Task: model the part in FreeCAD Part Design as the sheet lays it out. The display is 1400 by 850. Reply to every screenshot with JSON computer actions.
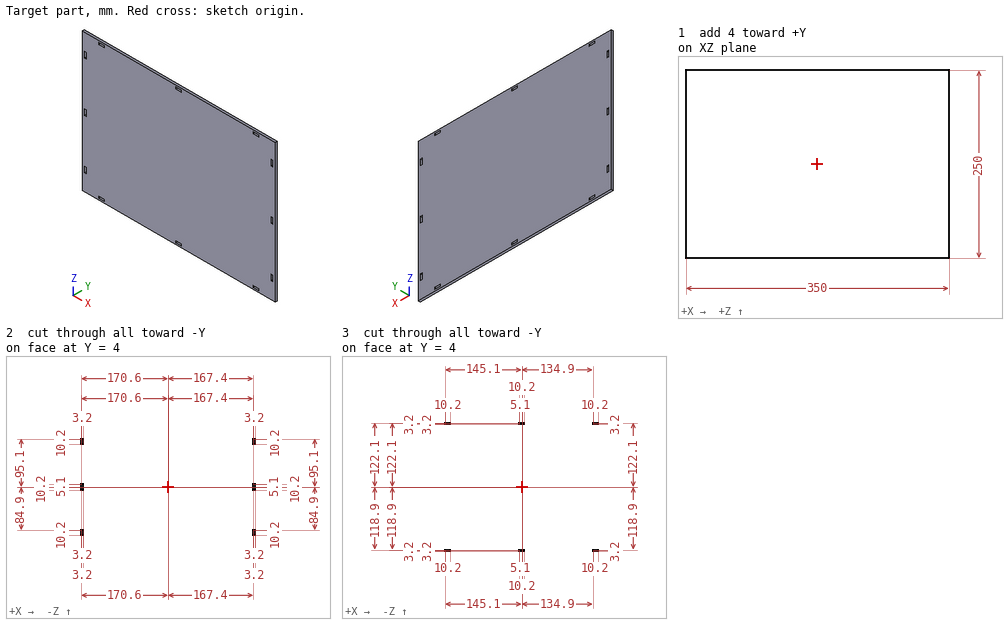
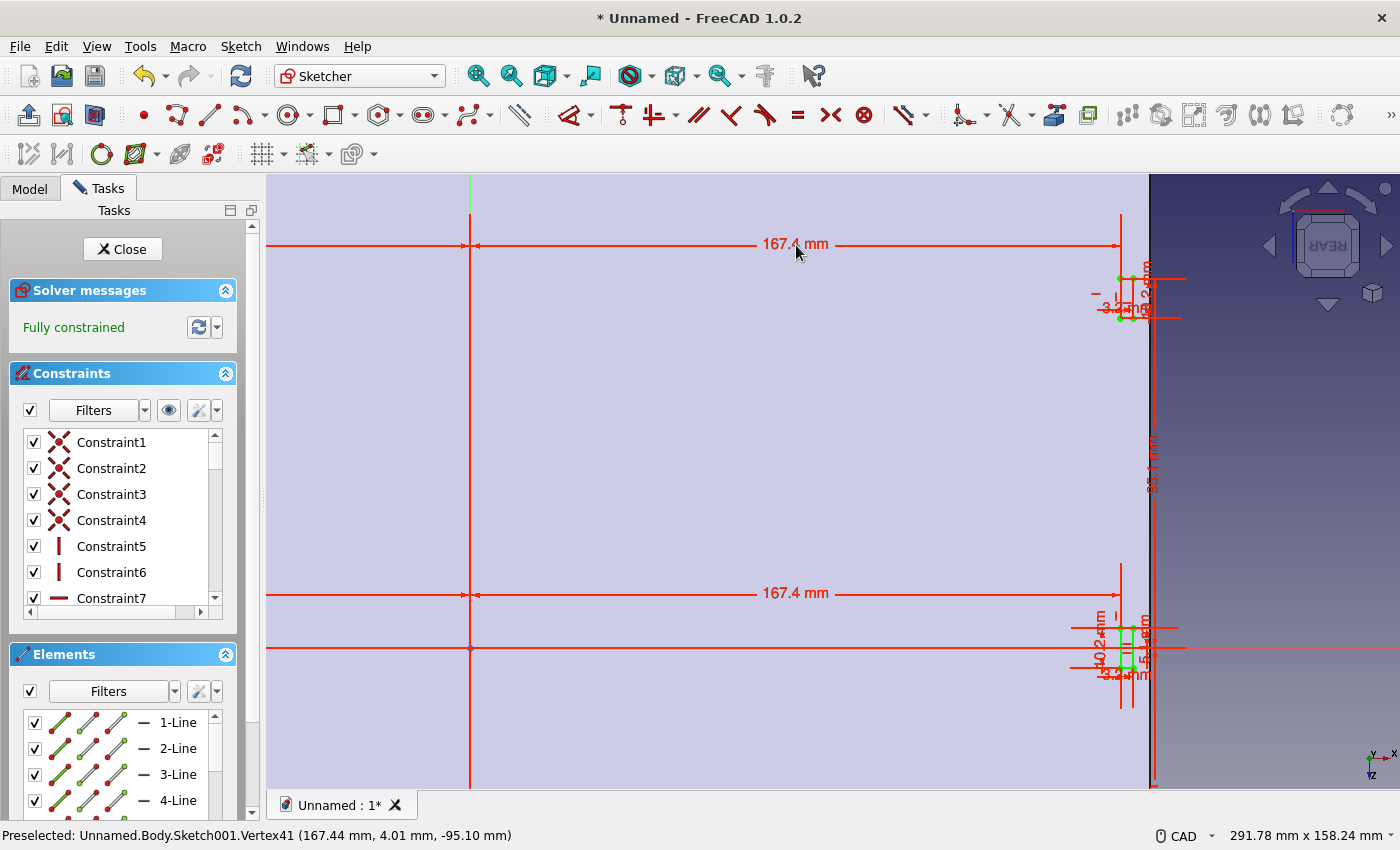
{"action": "left_click", "coordinate": [123, 249]}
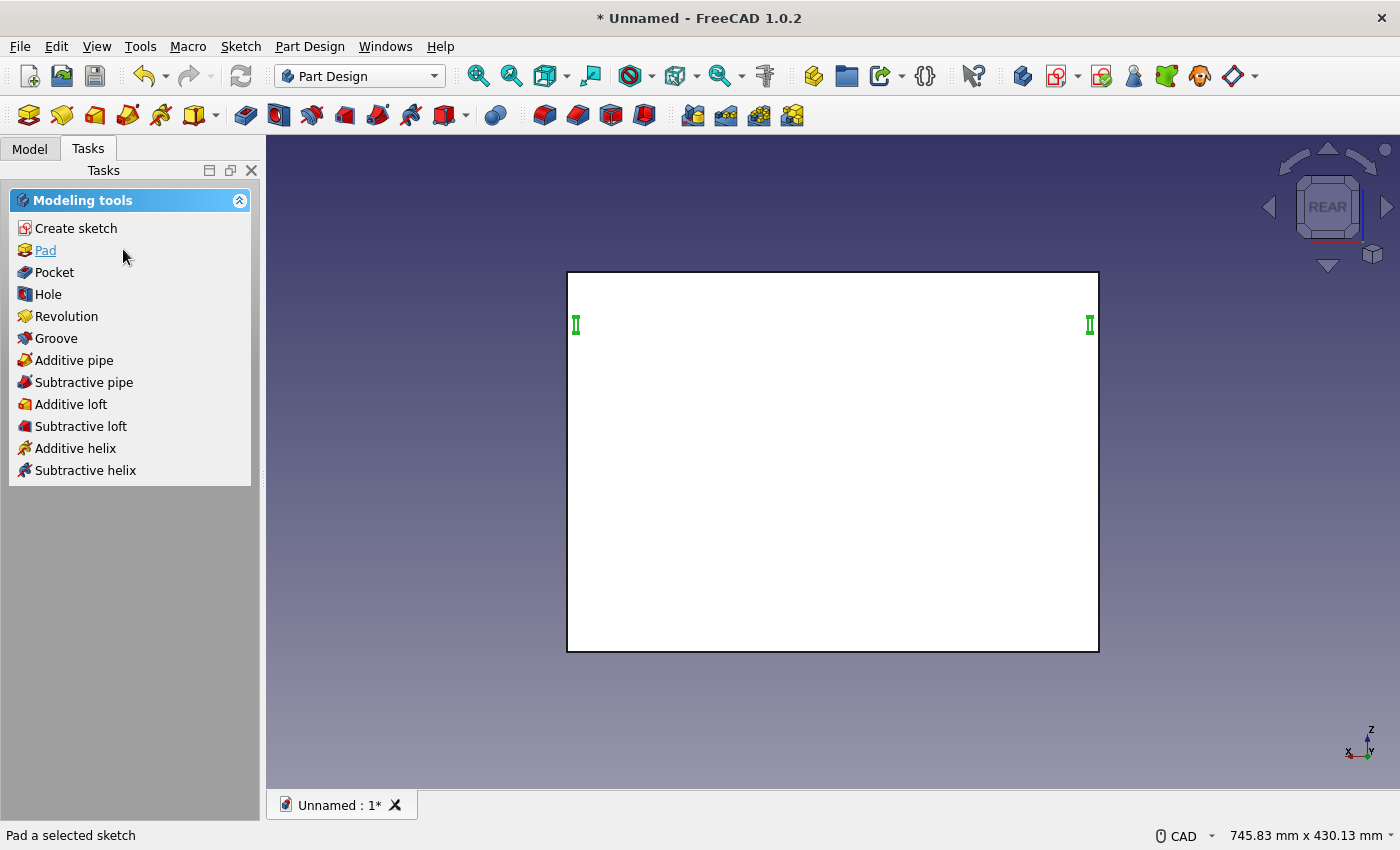
{"action": "left_click", "coordinate": [246, 116]}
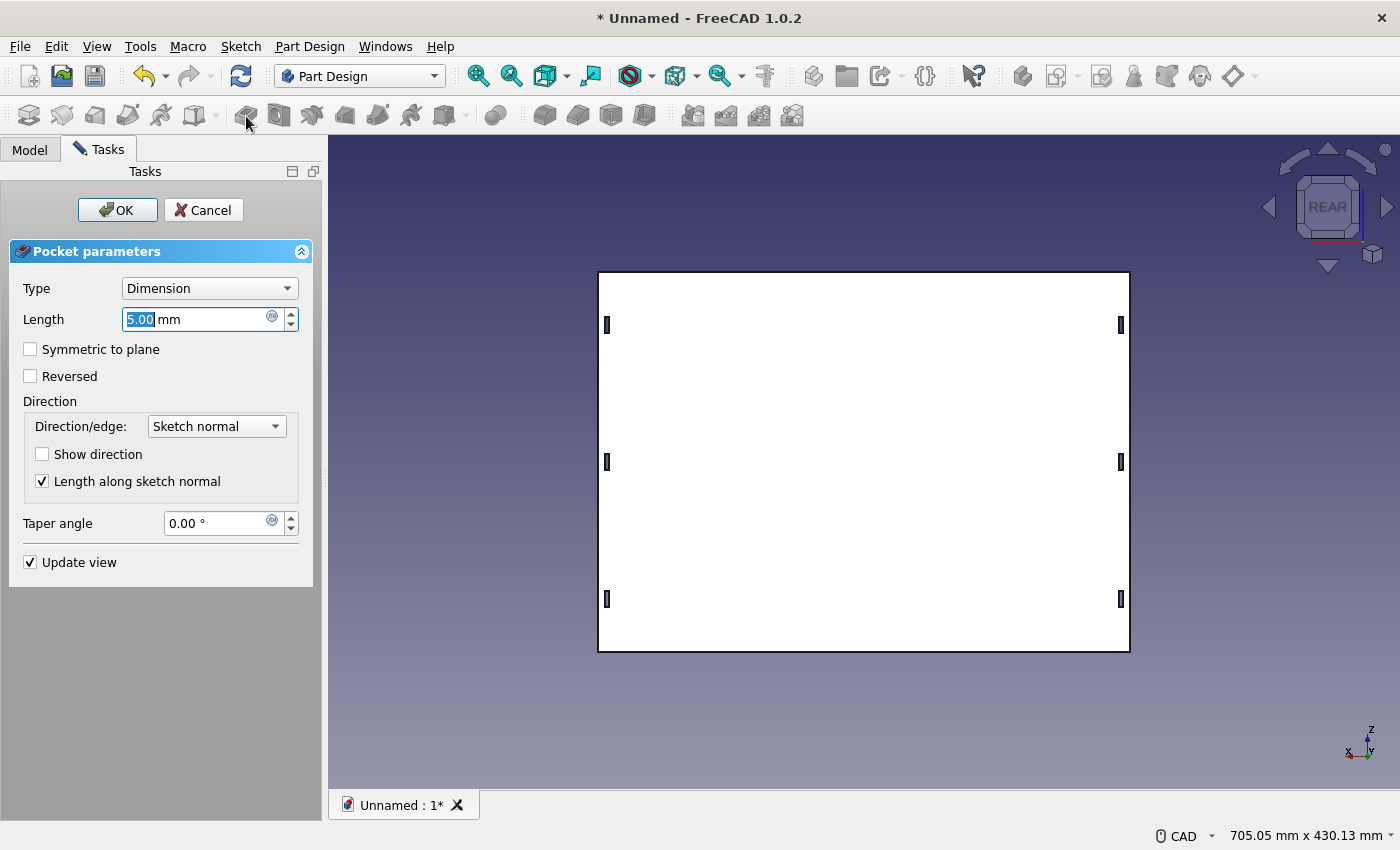
{"action": "left_click", "coordinate": [210, 288]}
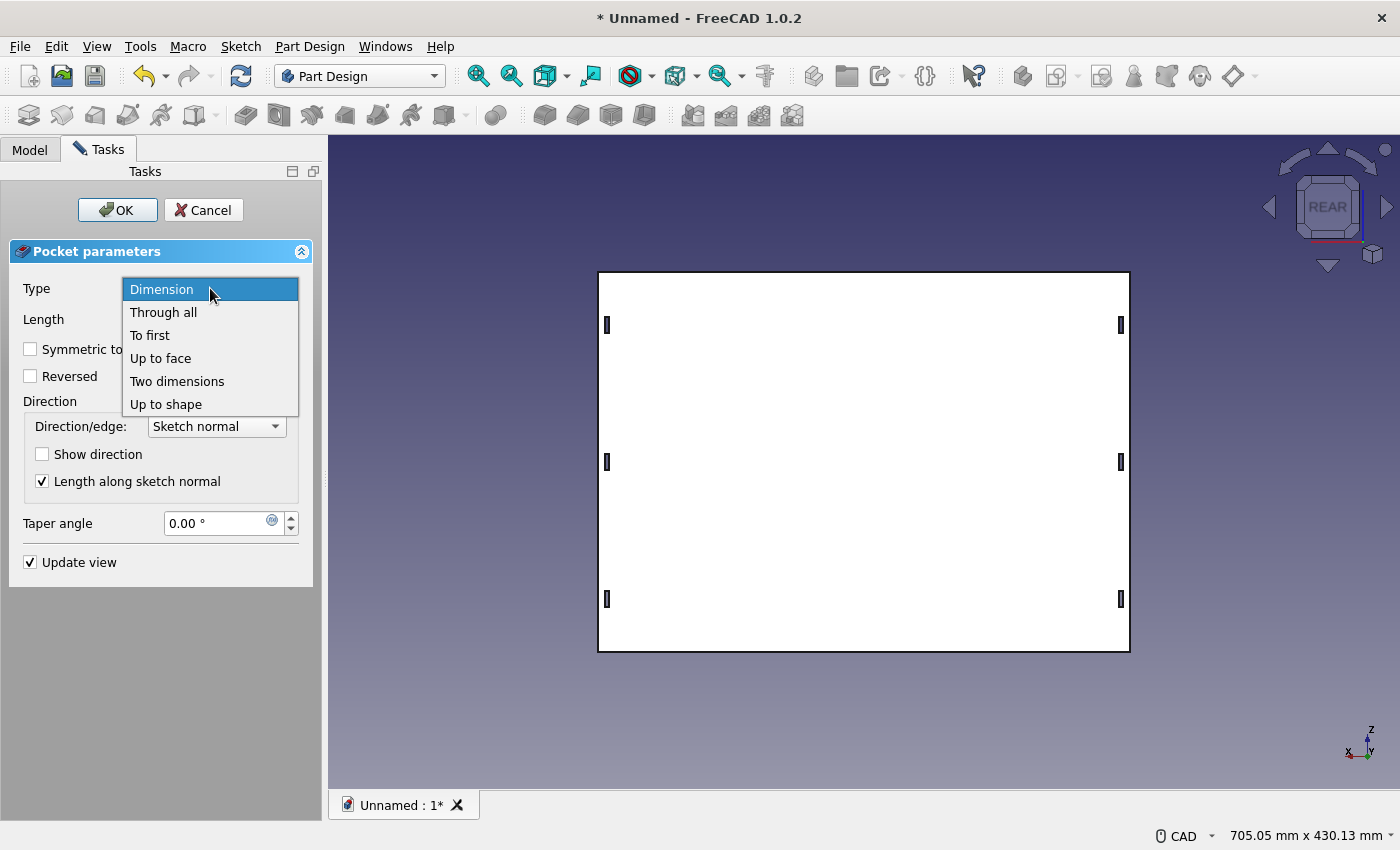
{"action": "left_click", "coordinate": [208, 312]}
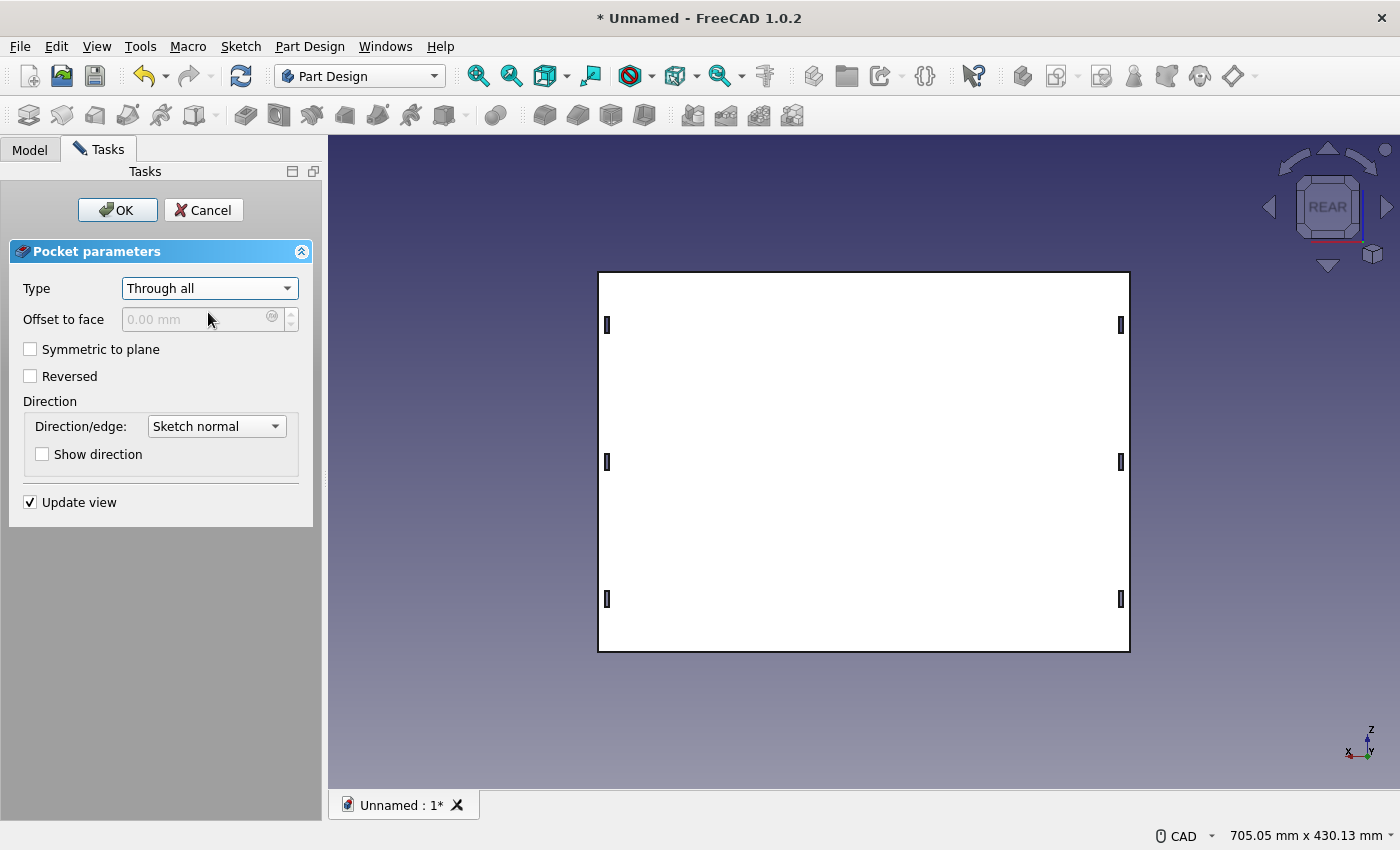
{"action": "left_click", "coordinate": [118, 210]}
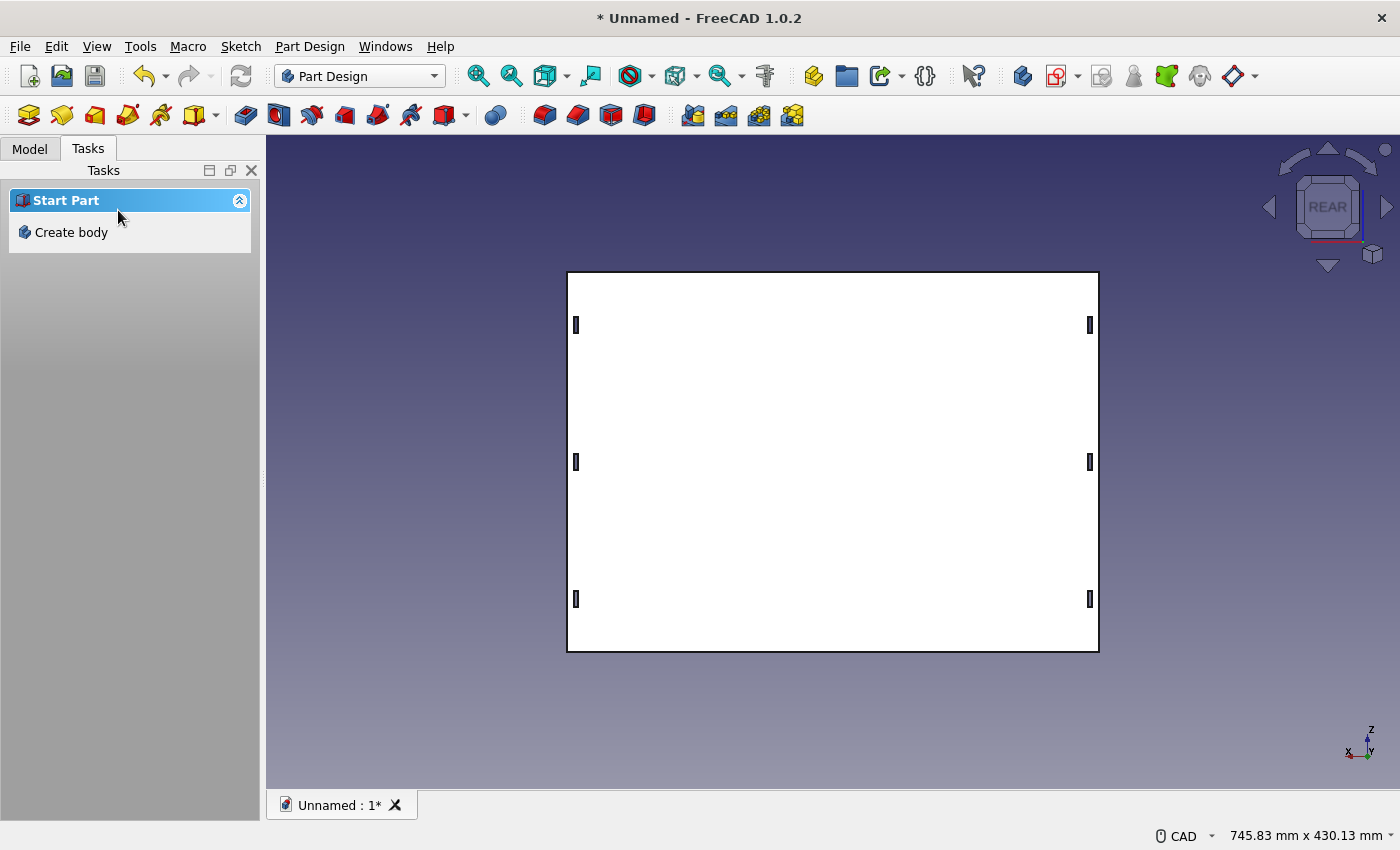
{"action": "left_click", "coordinate": [833, 461]}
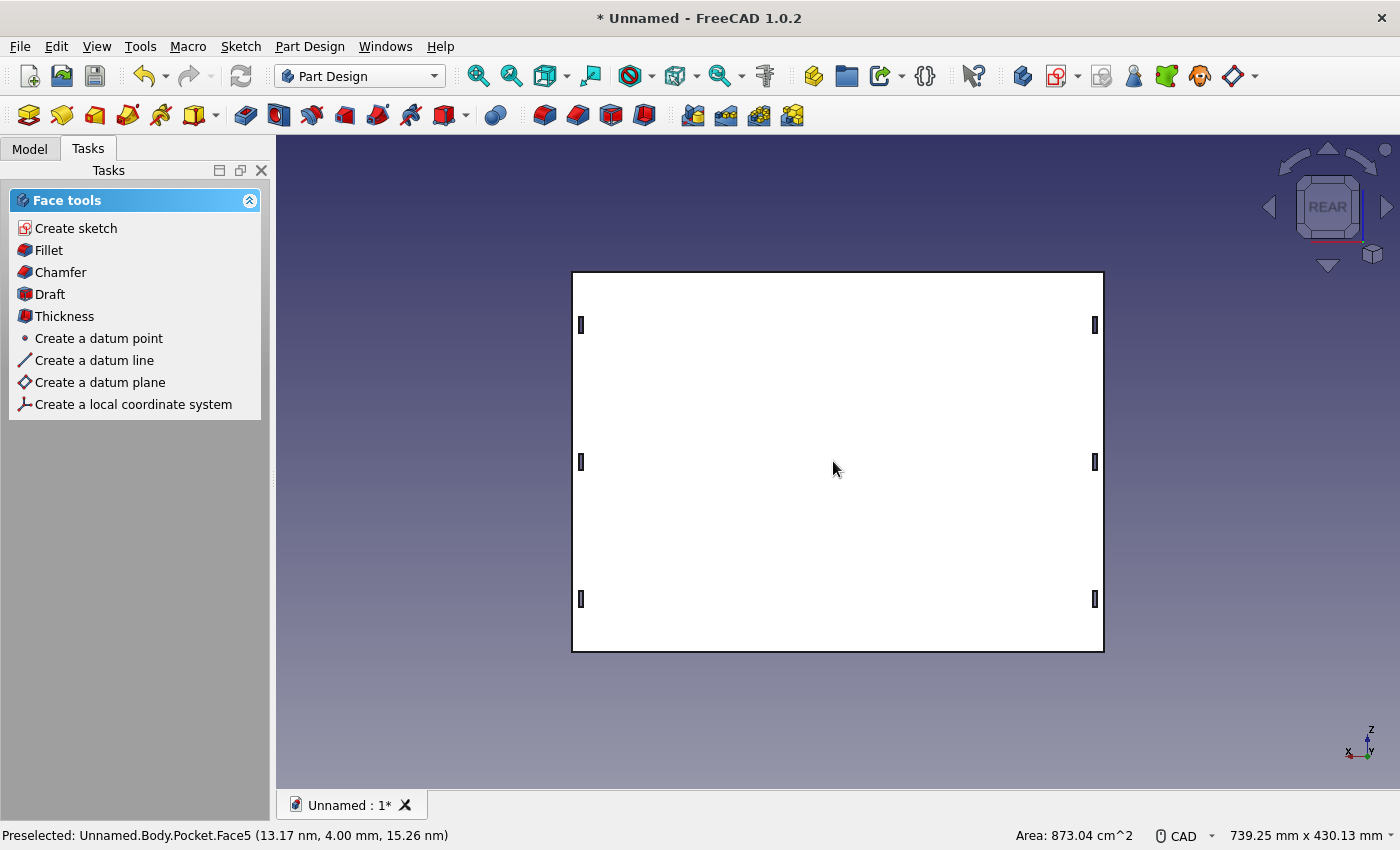
{"action": "left_click", "coordinate": [1056, 76]}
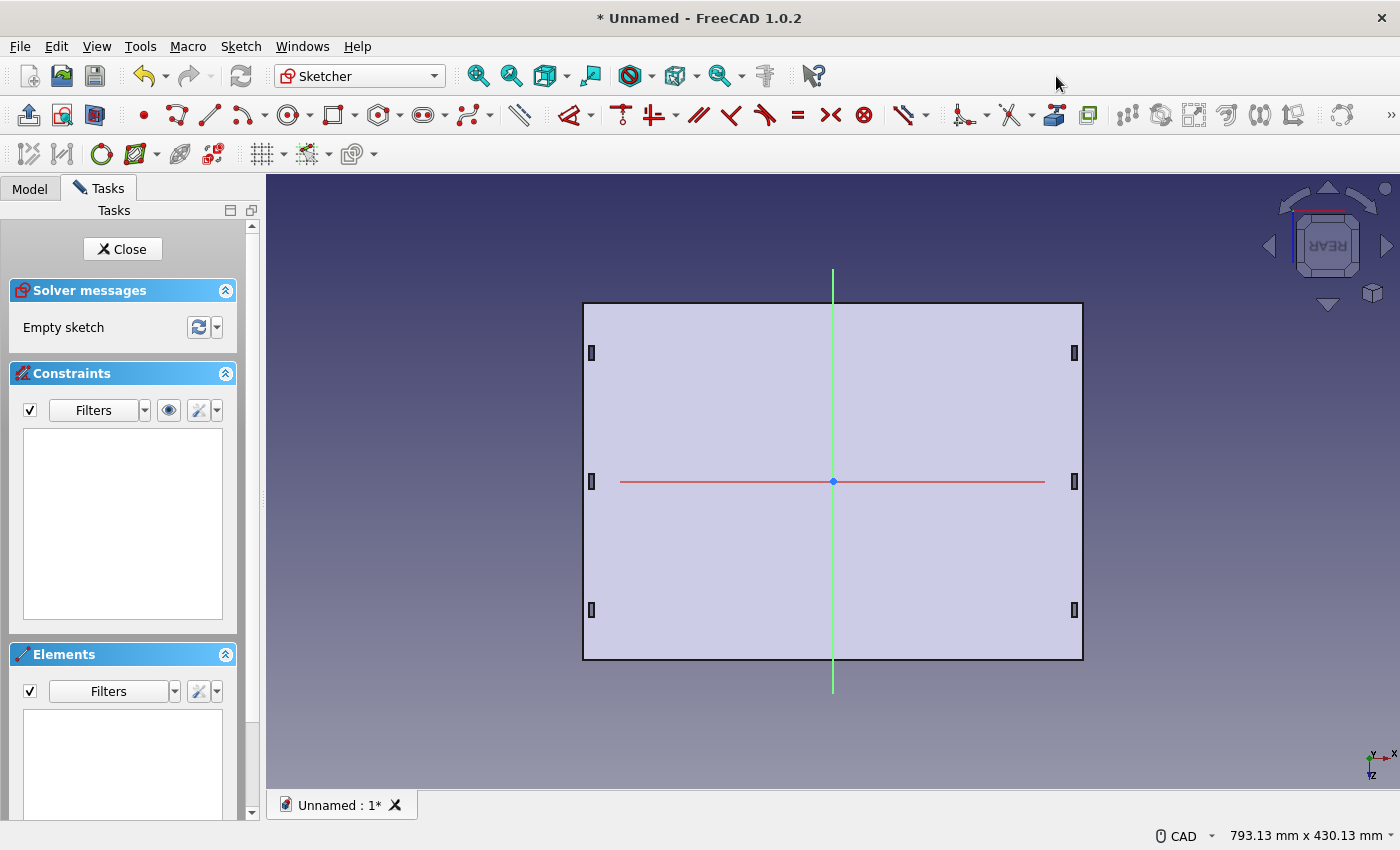
{"action": "left_click", "coordinate": [332, 116]}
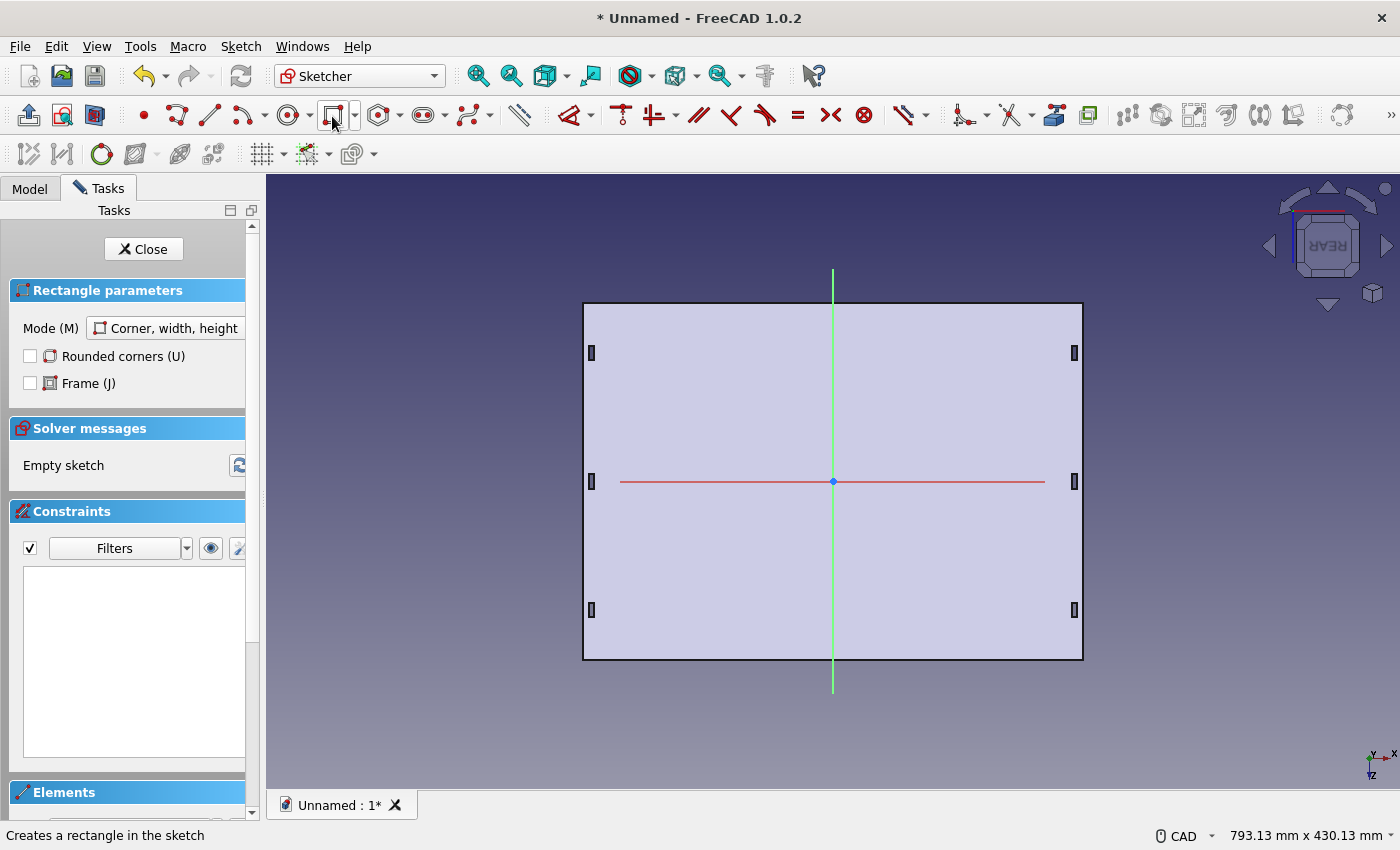
{"action": "scroll", "coordinate": [826, 307], "scroll_direction": "up", "scroll_amount": 7}